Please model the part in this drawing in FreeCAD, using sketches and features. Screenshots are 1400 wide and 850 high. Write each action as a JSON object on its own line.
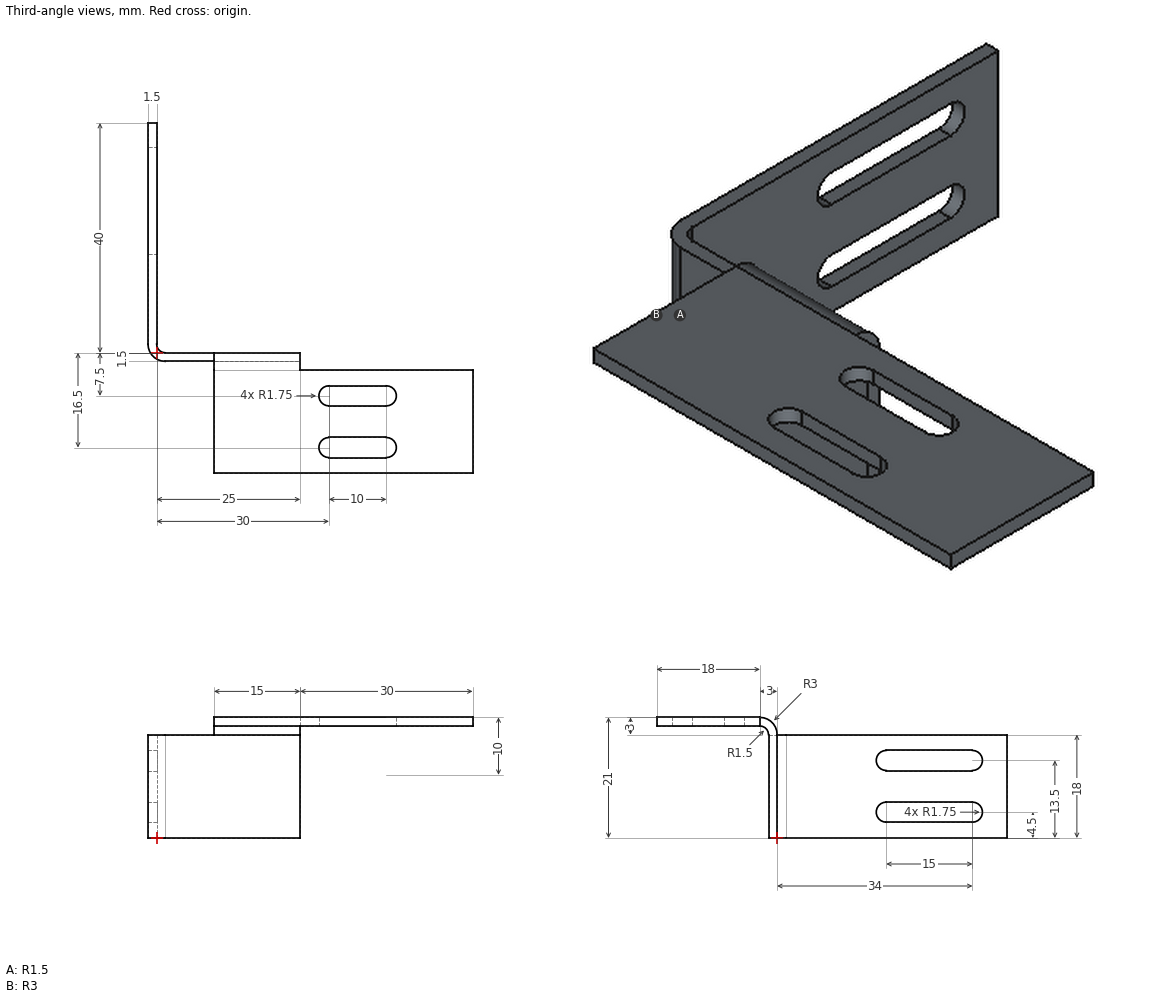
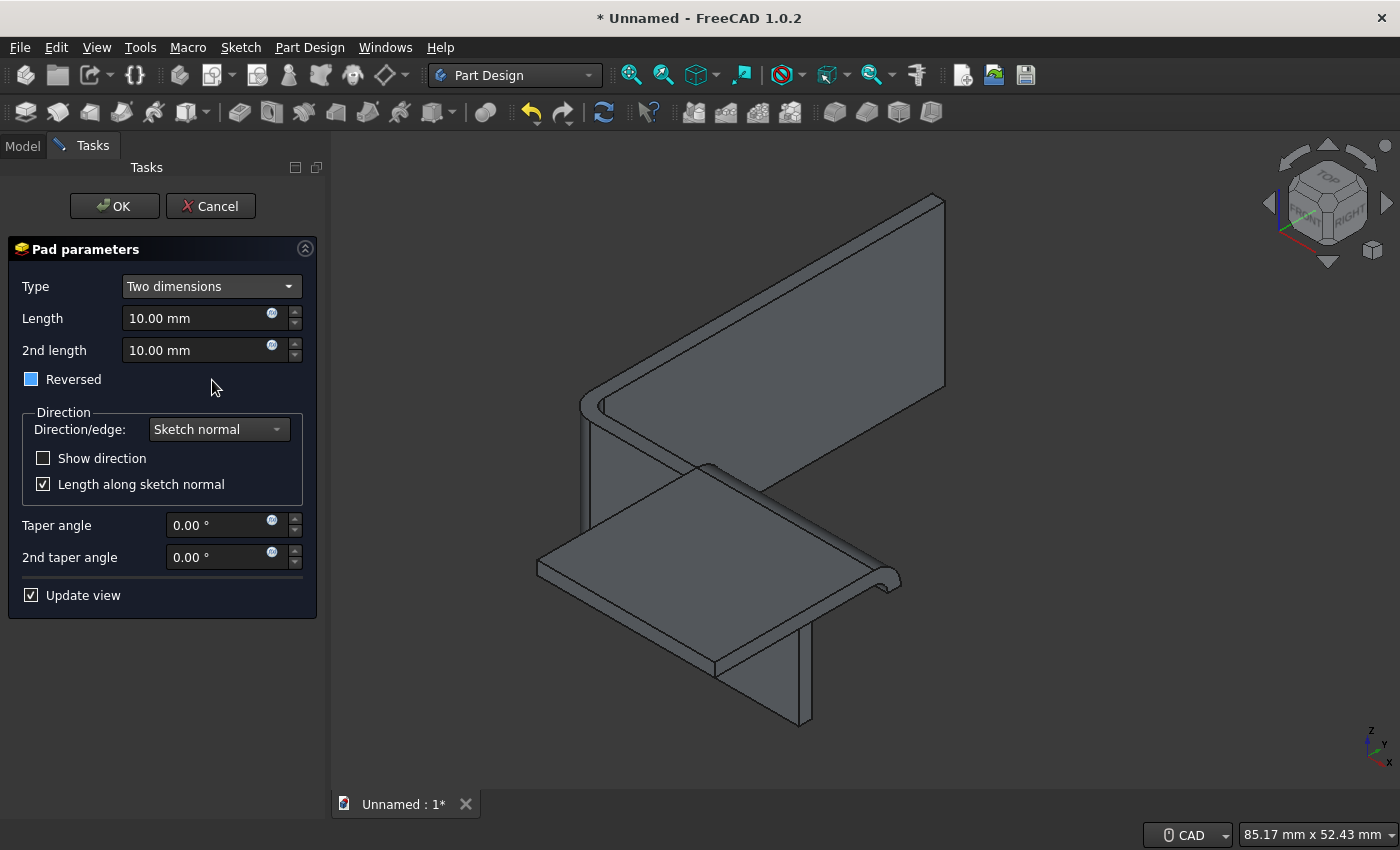
{"action": "triple_click", "coordinate": [204, 318]}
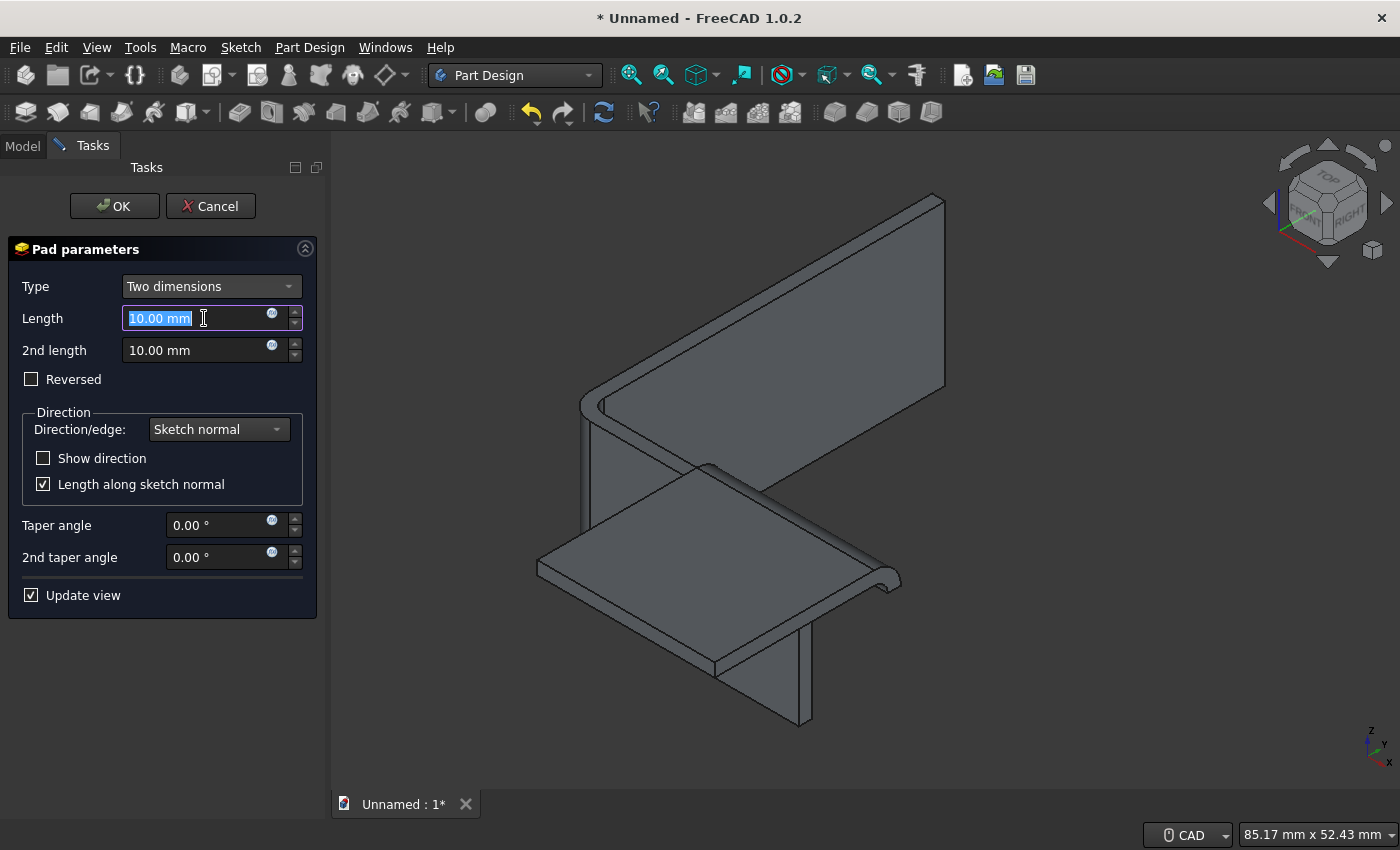
{"action": "type", "text": "30"}
{"action": "key", "text": "Tab"}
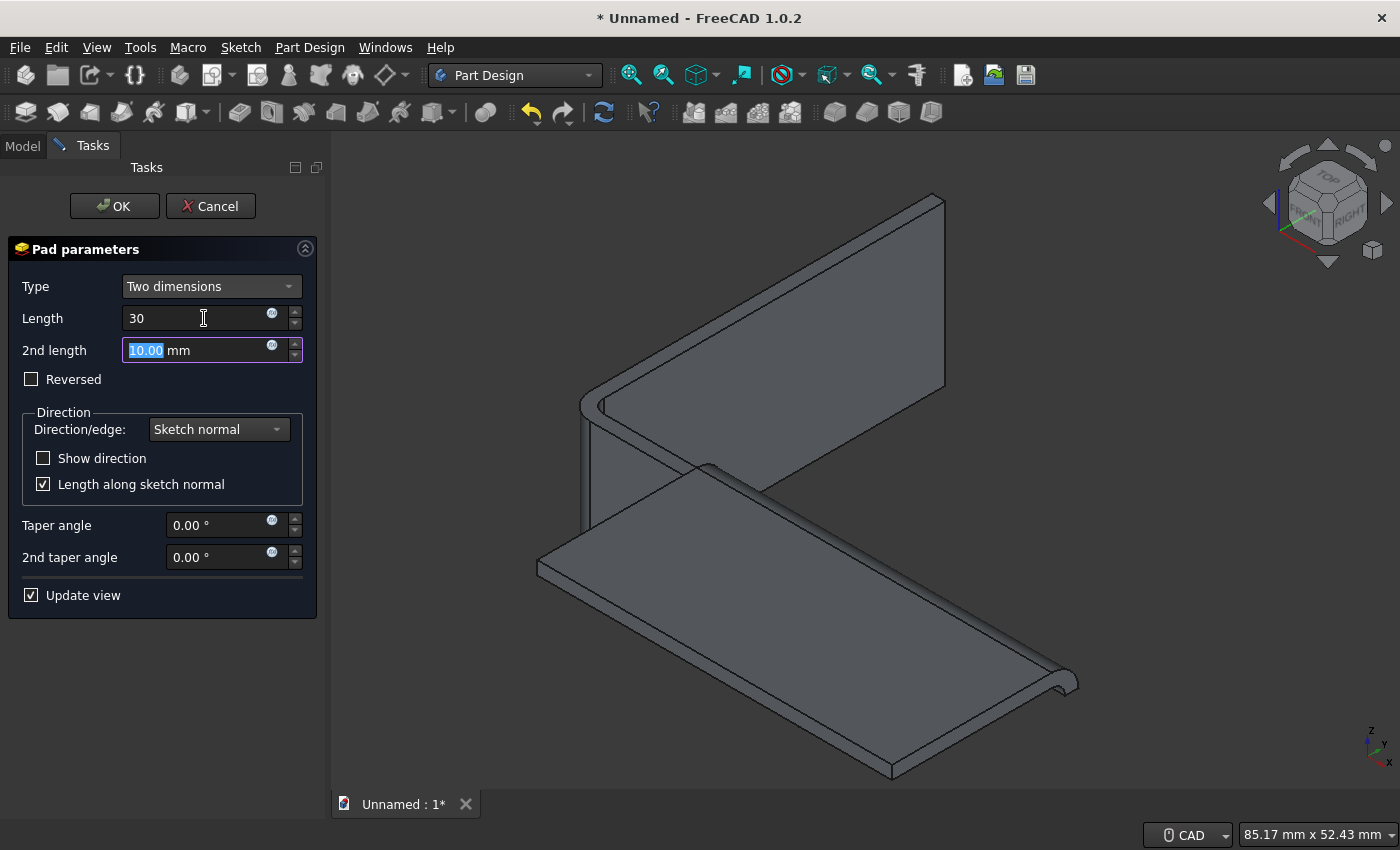
{"action": "type", "text": "15"}
{"action": "key", "text": "Tab"}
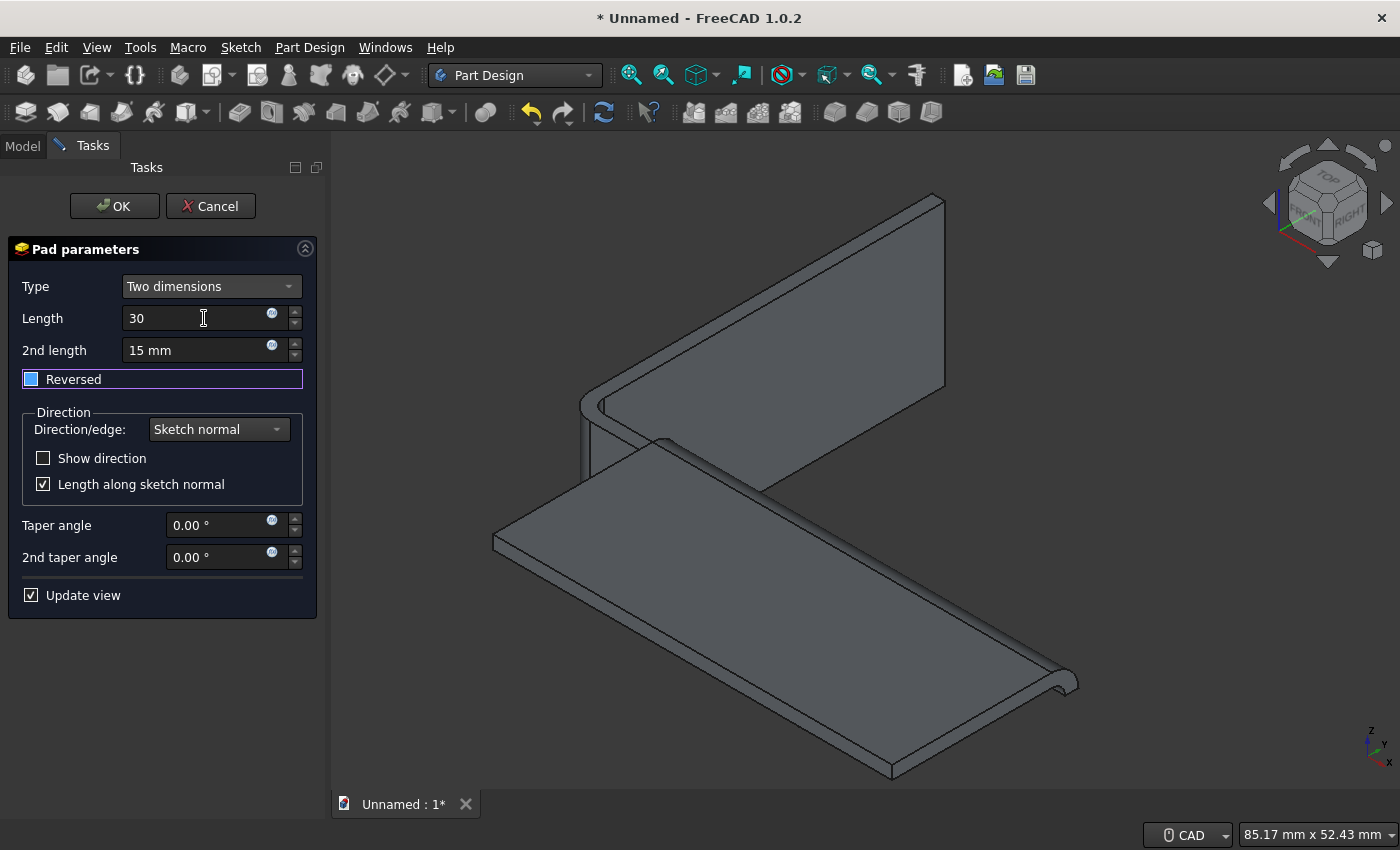
{"action": "left_click", "coordinate": [115, 206]}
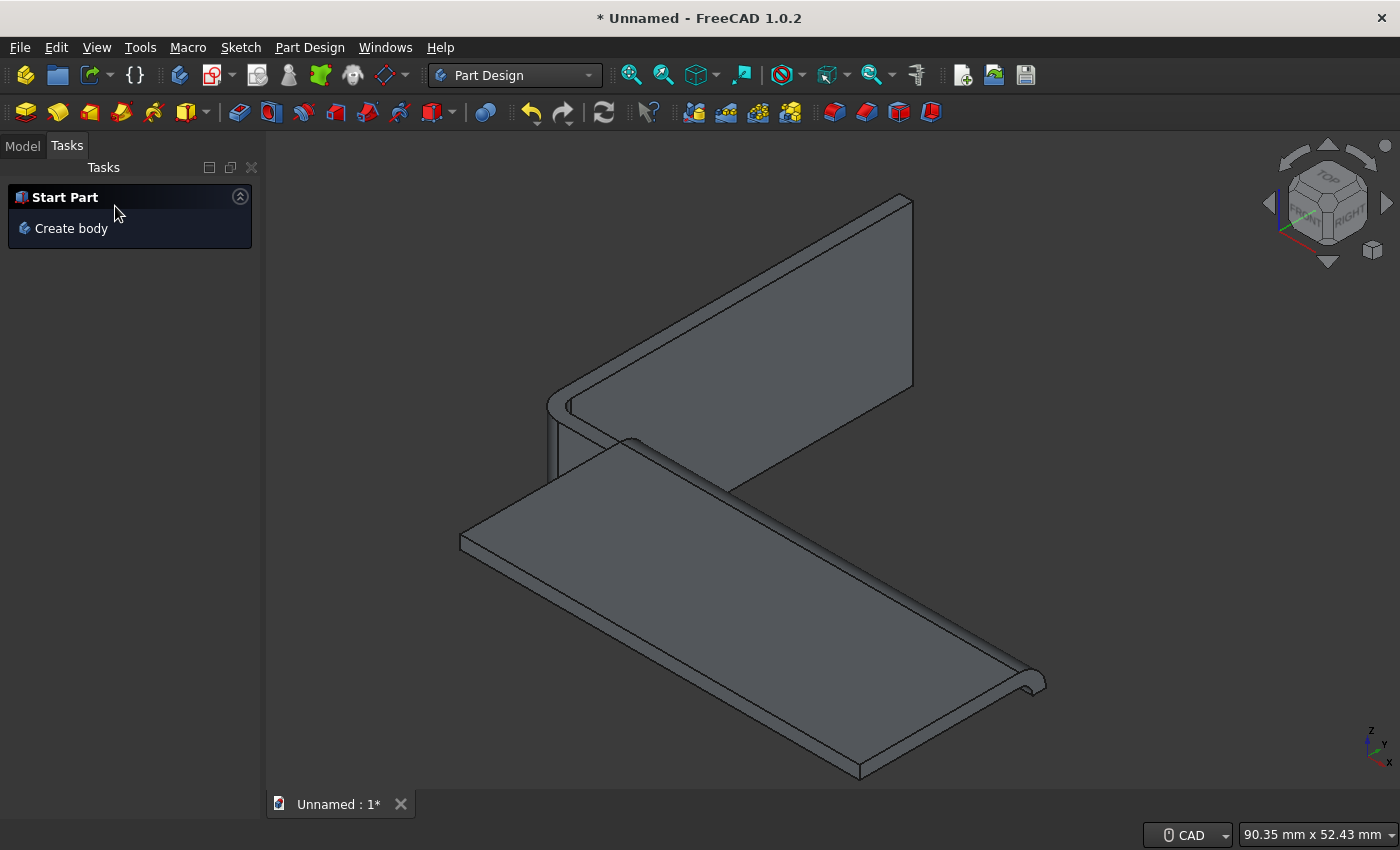
{"action": "left_click", "coordinate": [632, 76]}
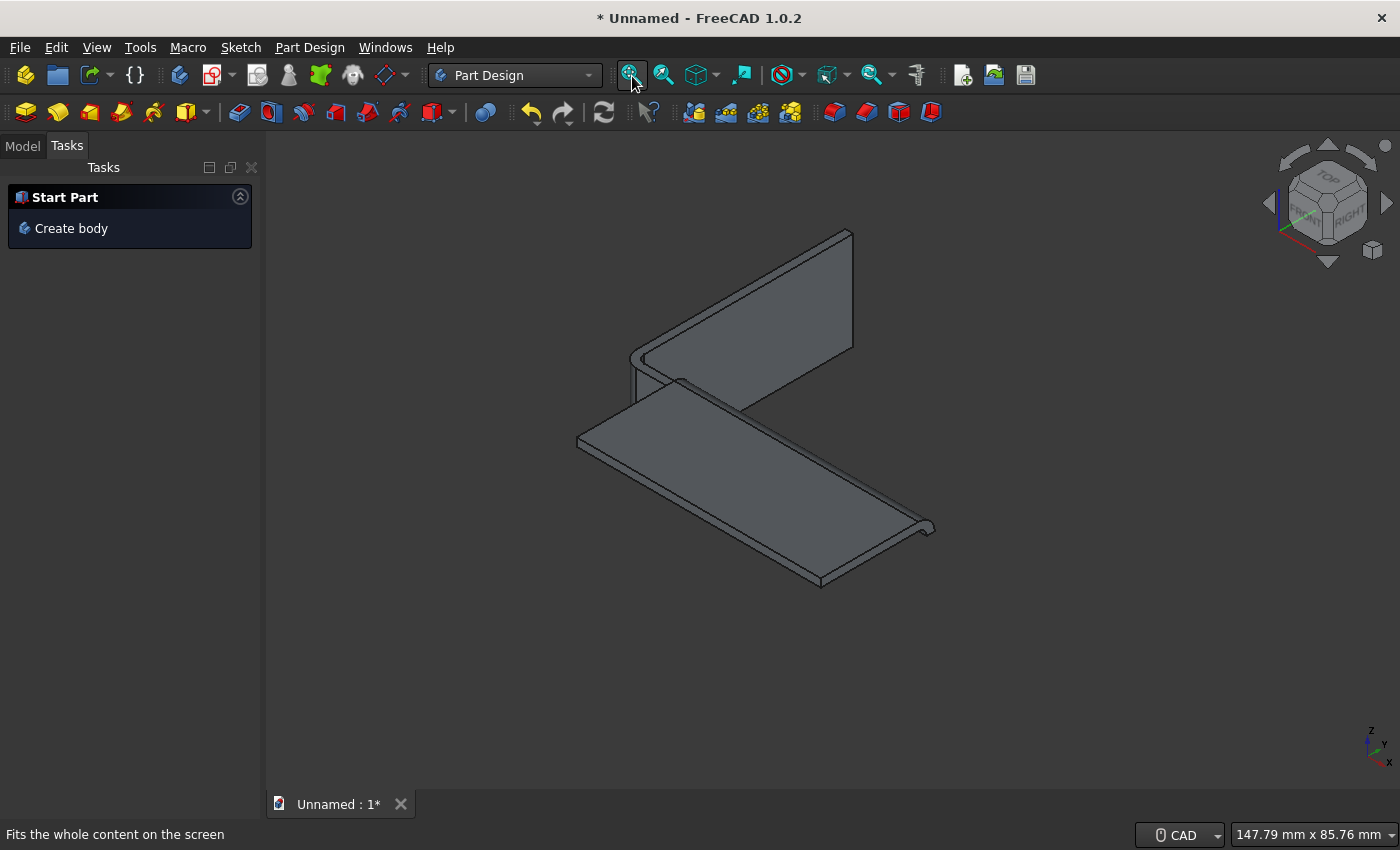
{"action": "scroll", "coordinate": [910, 530], "scroll_direction": "up", "scroll_amount": 5}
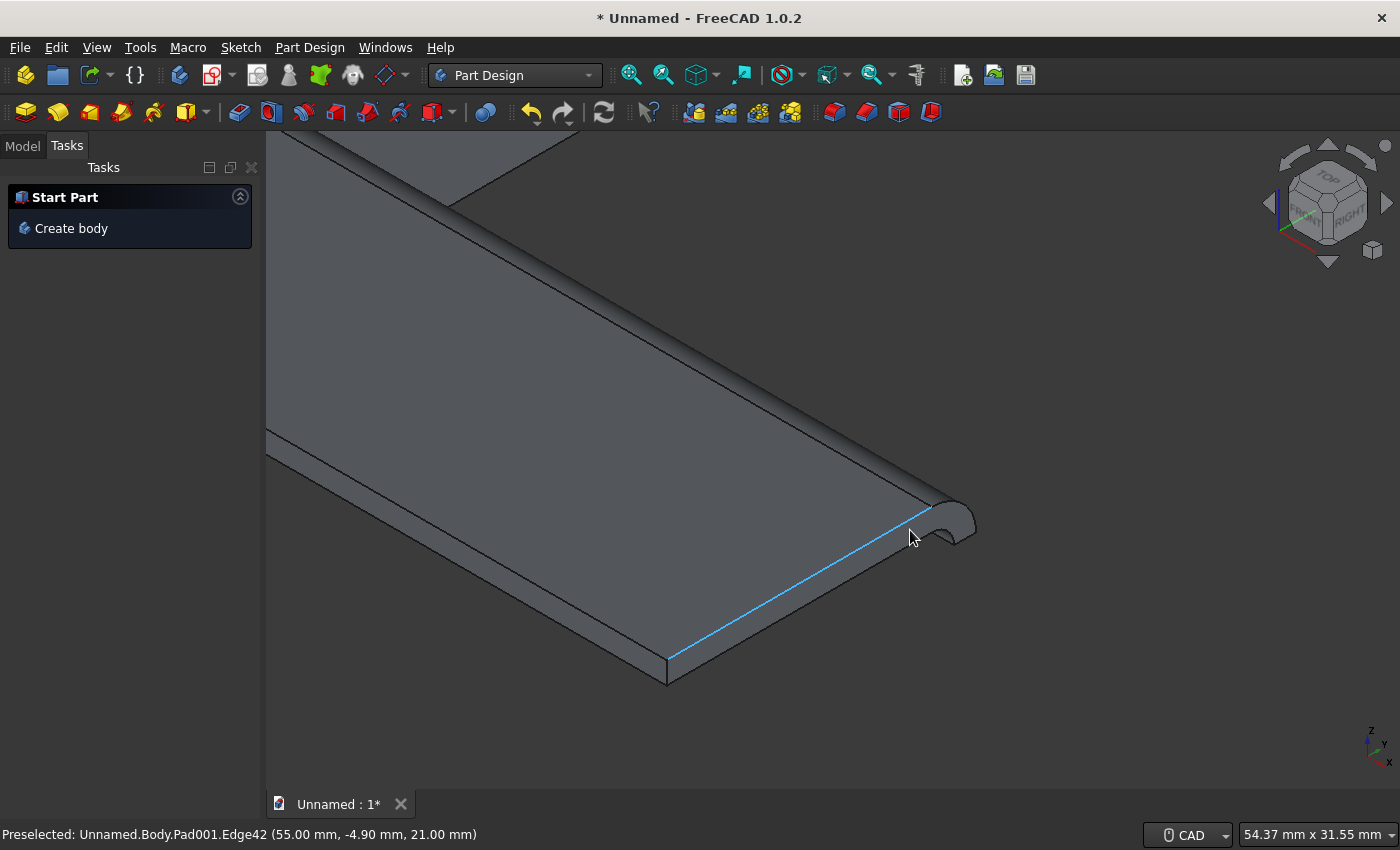
{"action": "left_click", "coordinate": [910, 530]}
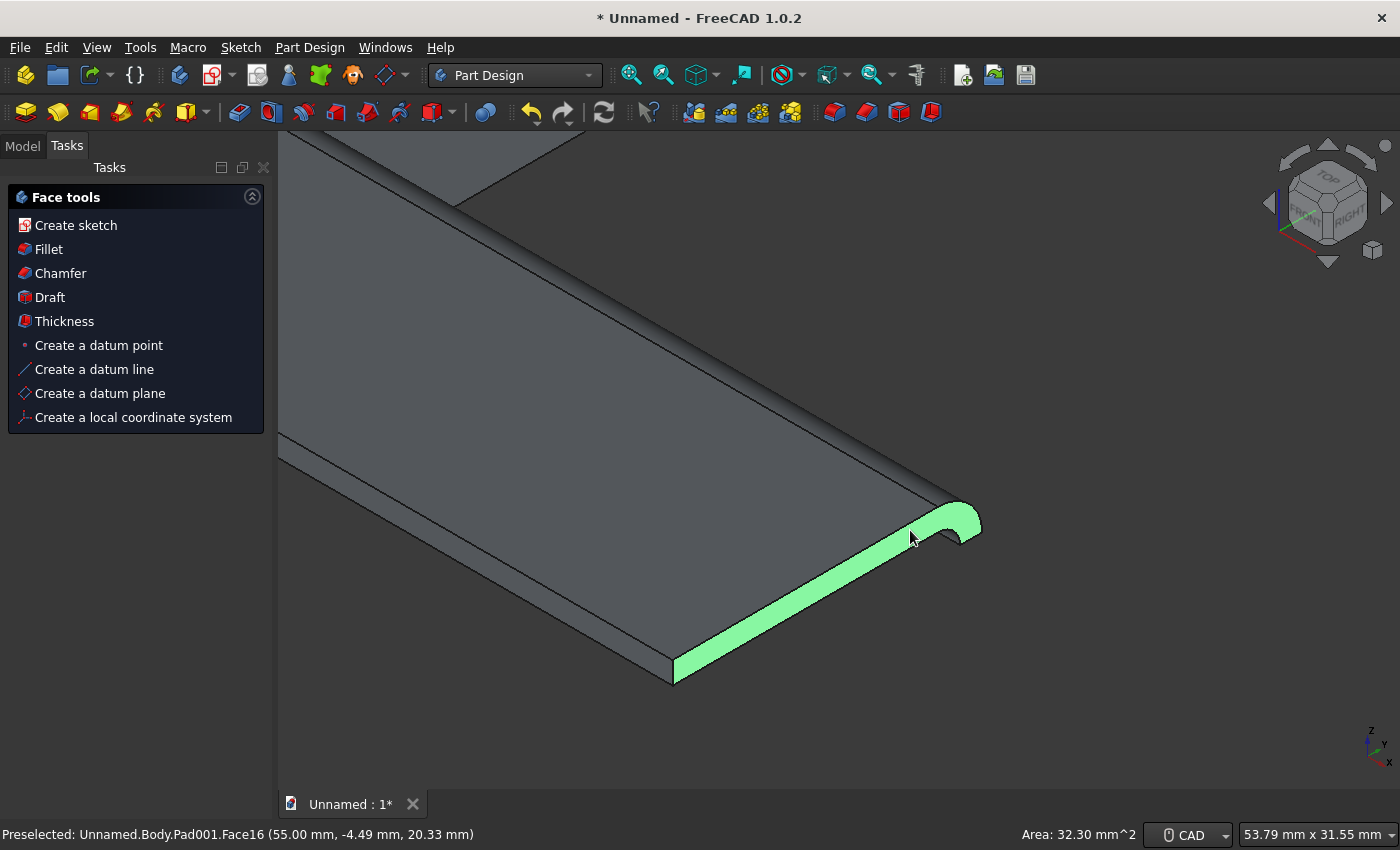
{"action": "left_click", "coordinate": [212, 76]}